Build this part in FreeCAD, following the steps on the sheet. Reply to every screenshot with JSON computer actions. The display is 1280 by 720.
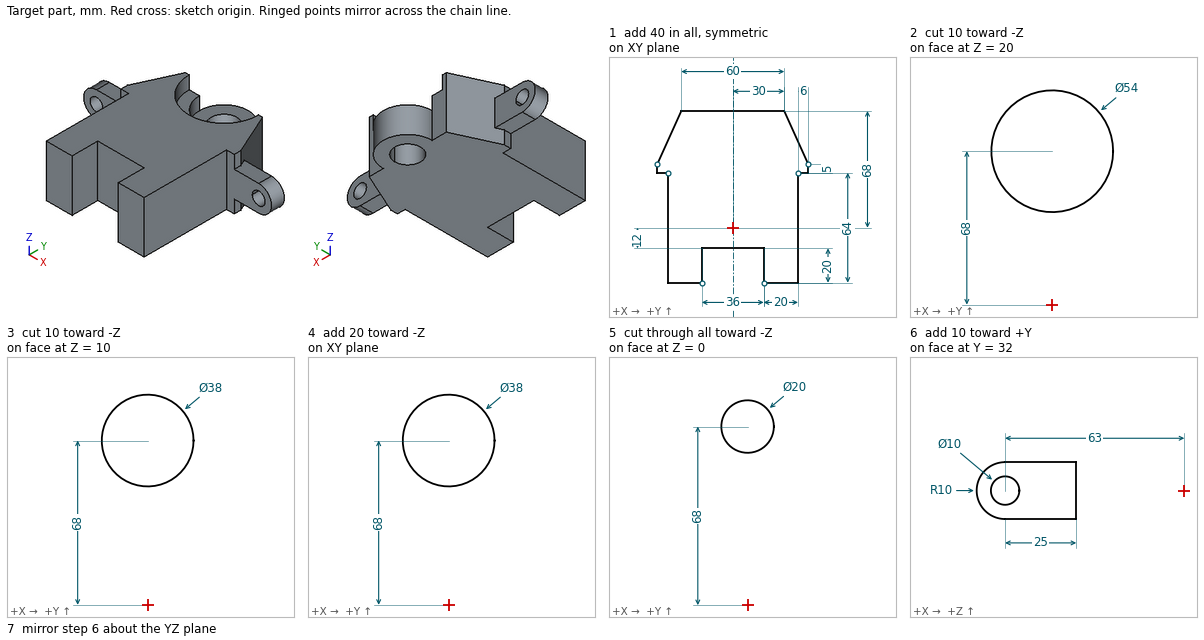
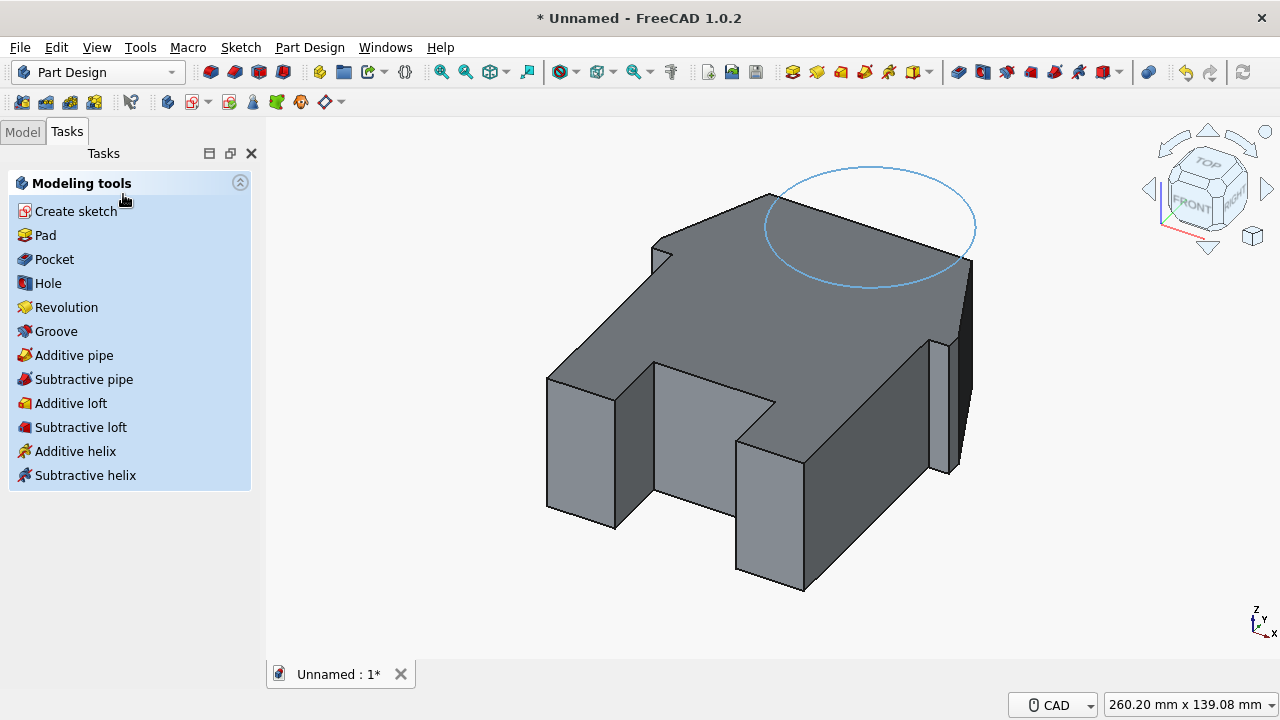
{"action": "left_click", "coordinate": [960, 72]}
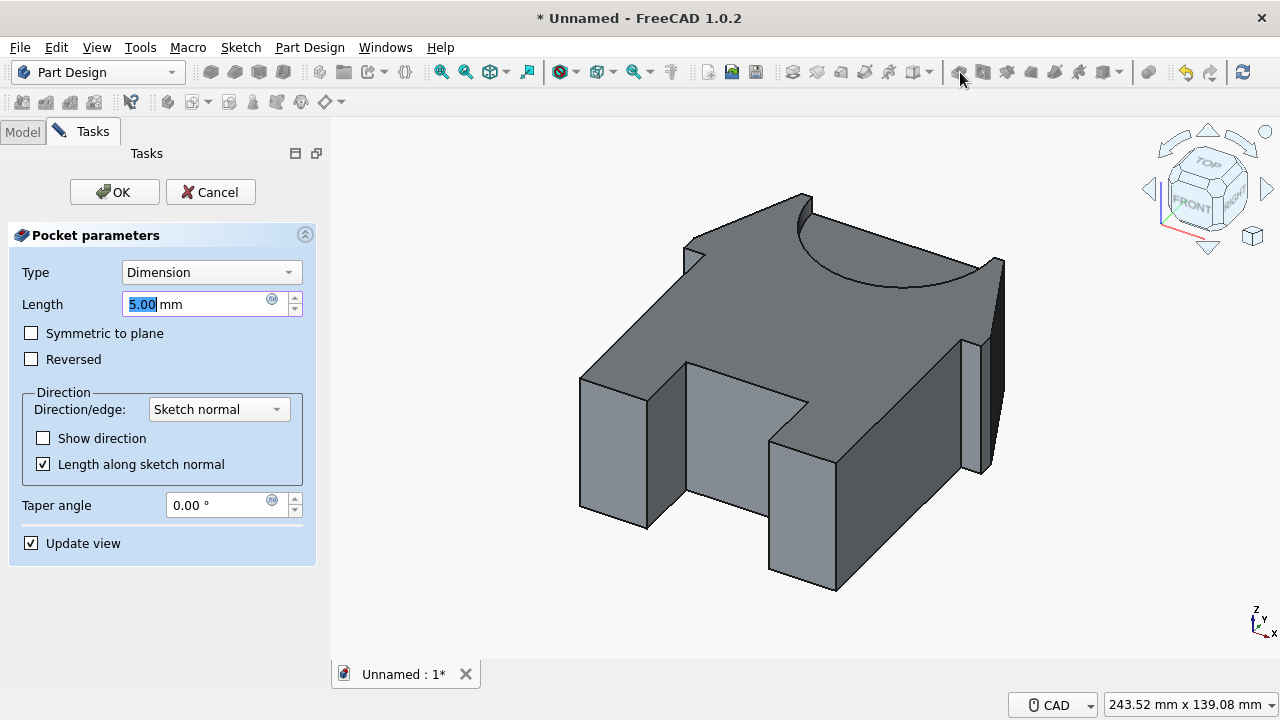
{"action": "type", "text": "10"}
{"action": "key", "text": "Tab"}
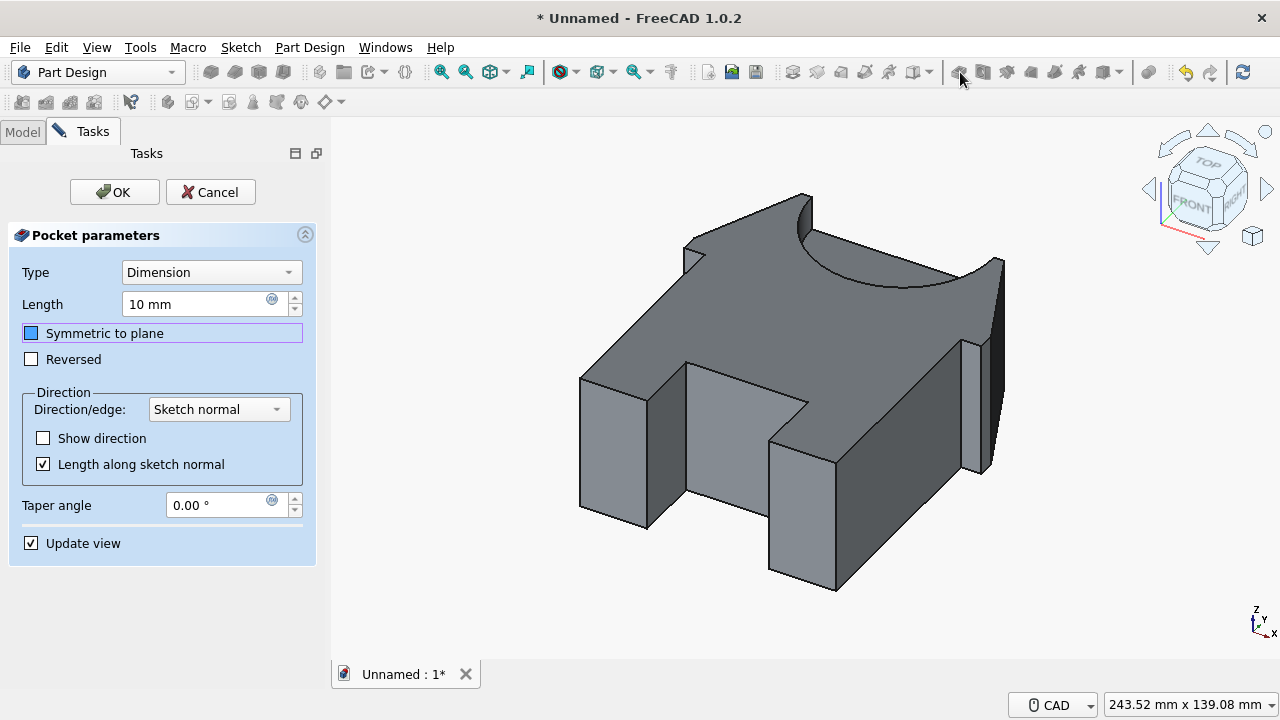
{"action": "left_click", "coordinate": [115, 192]}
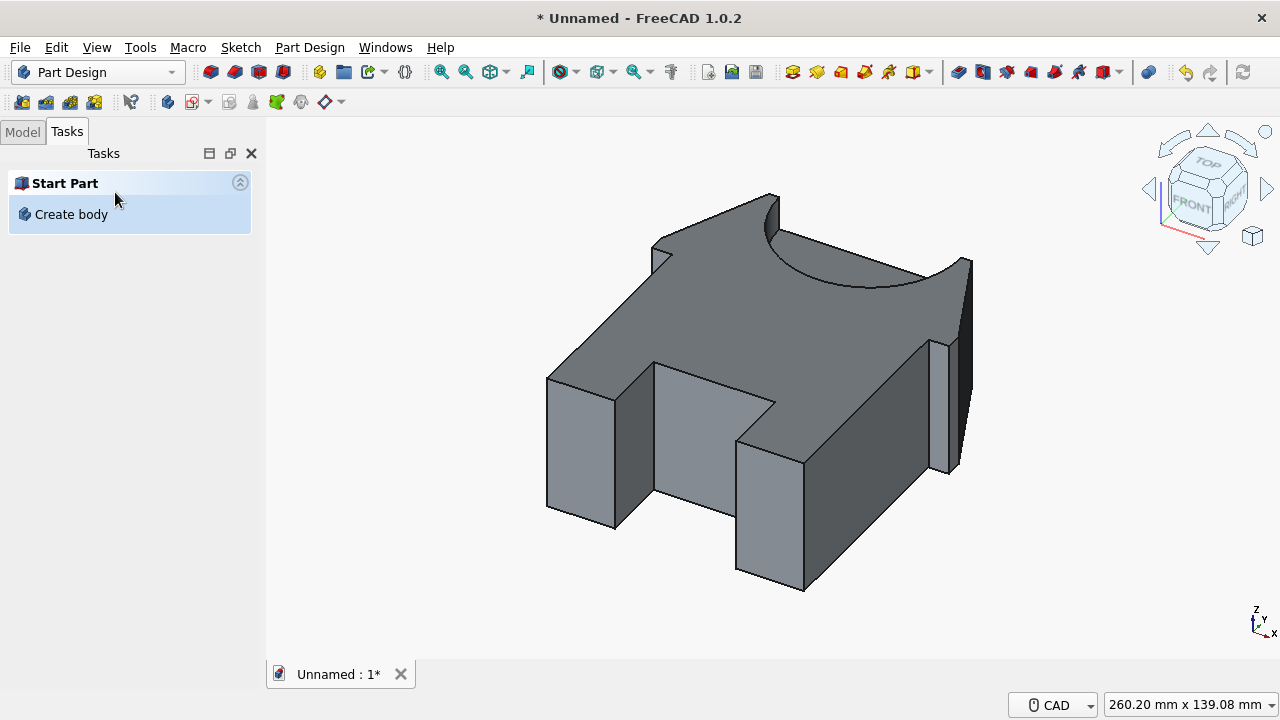
{"action": "left_click", "coordinate": [852, 277]}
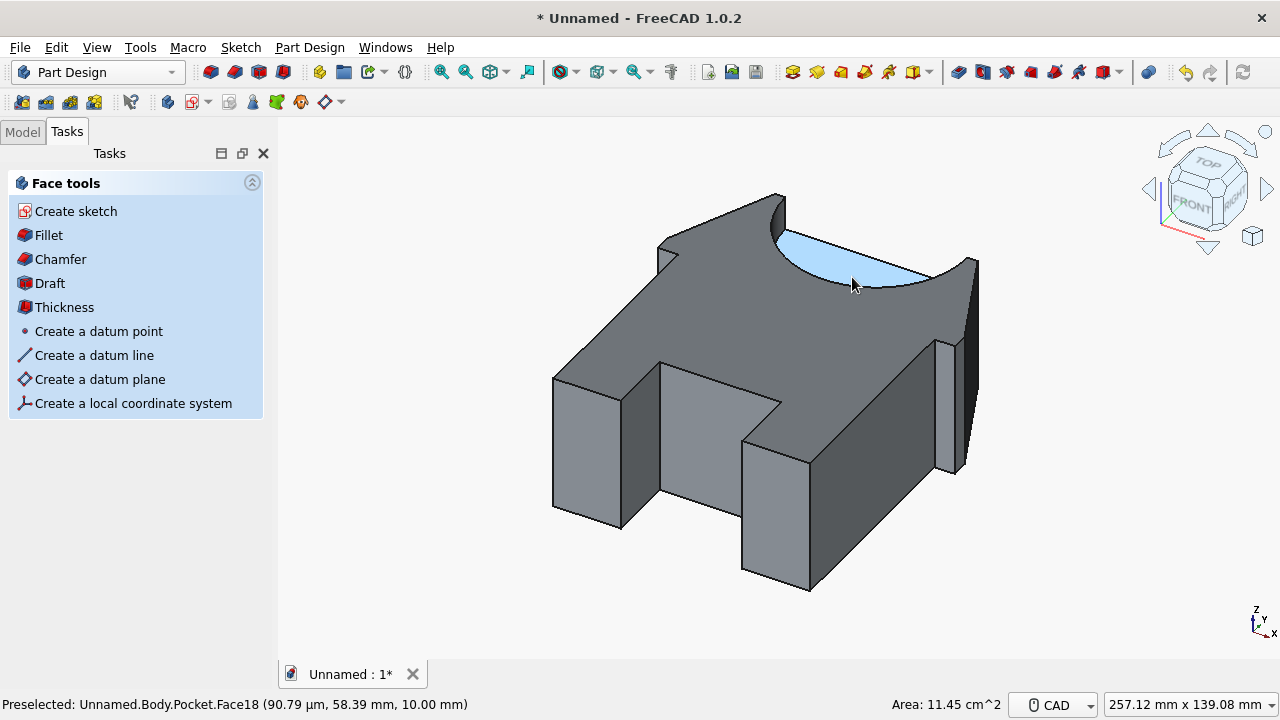
{"action": "left_click", "coordinate": [192, 102]}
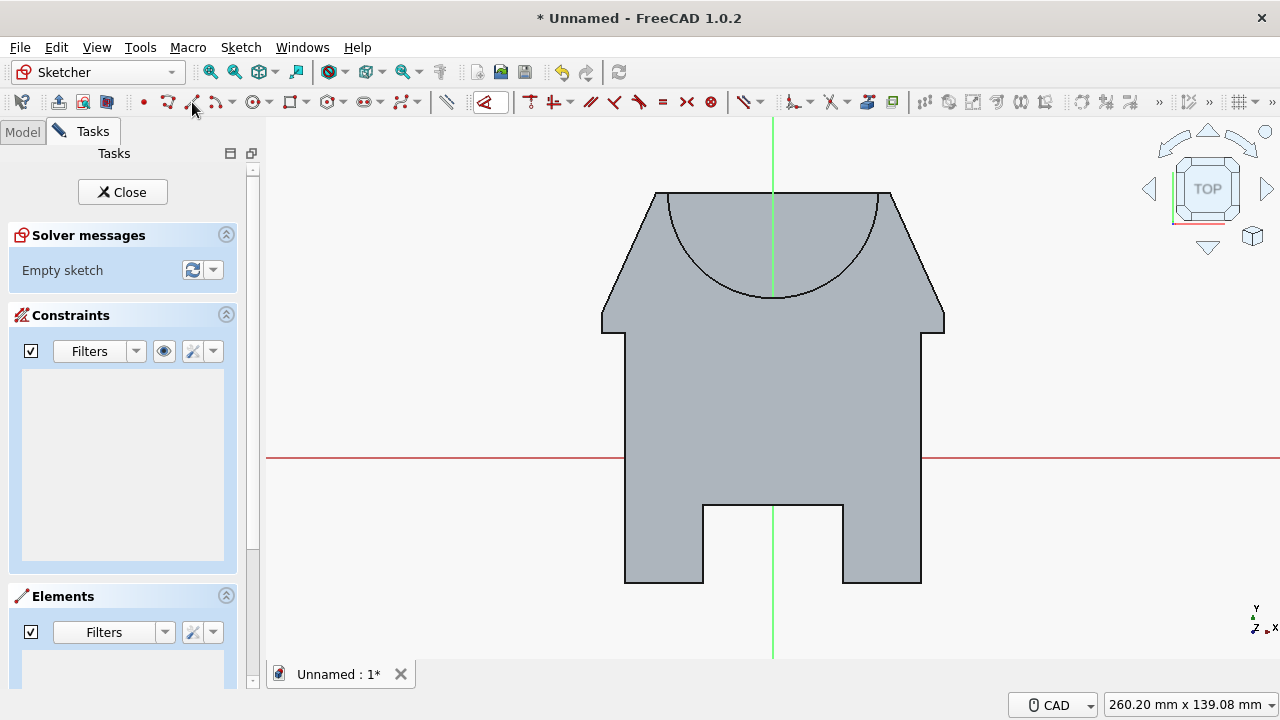
{"action": "left_click", "coordinate": [108, 102]}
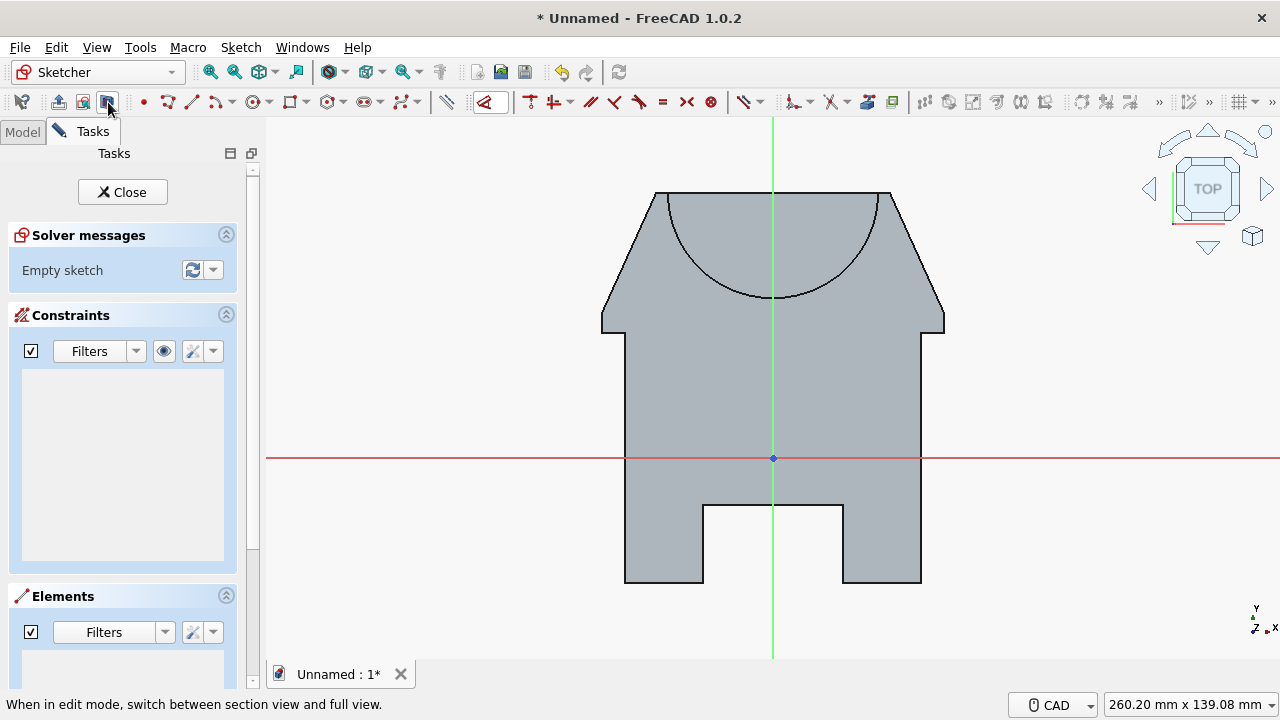
{"action": "scroll", "coordinate": [395, 631], "scroll_direction": "down", "scroll_amount": 1}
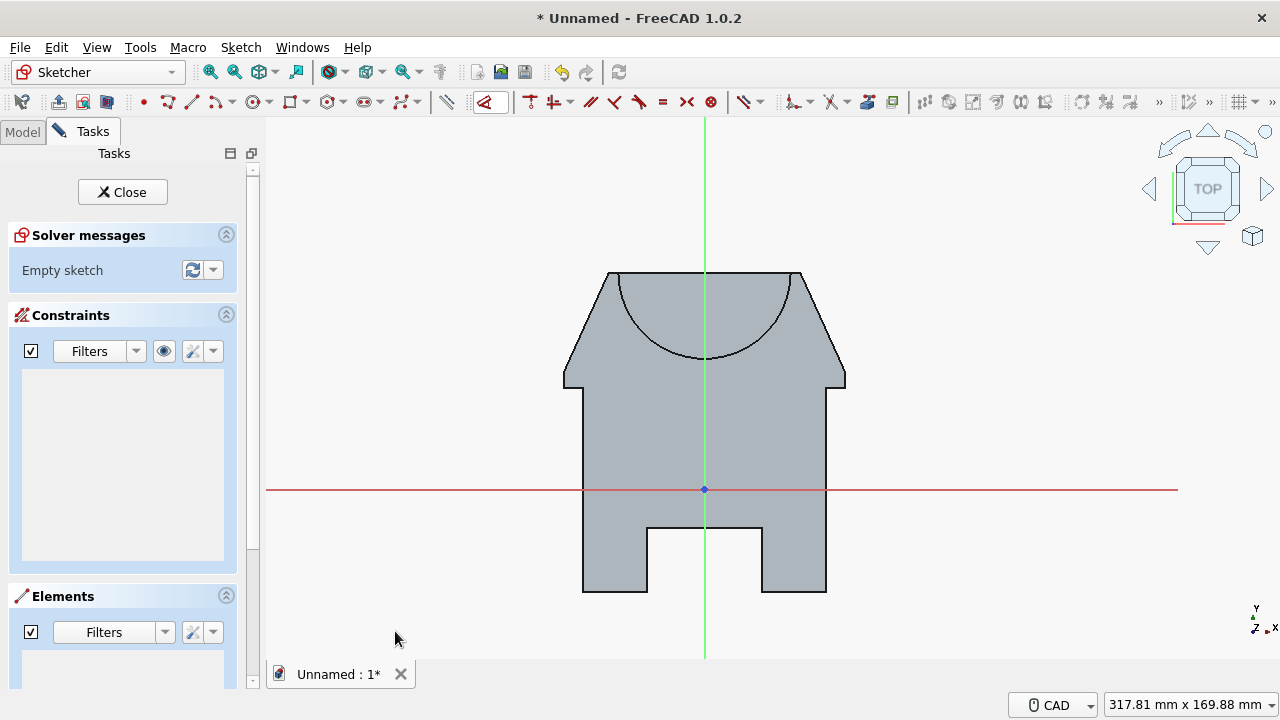
{"action": "left_click", "coordinate": [254, 102]}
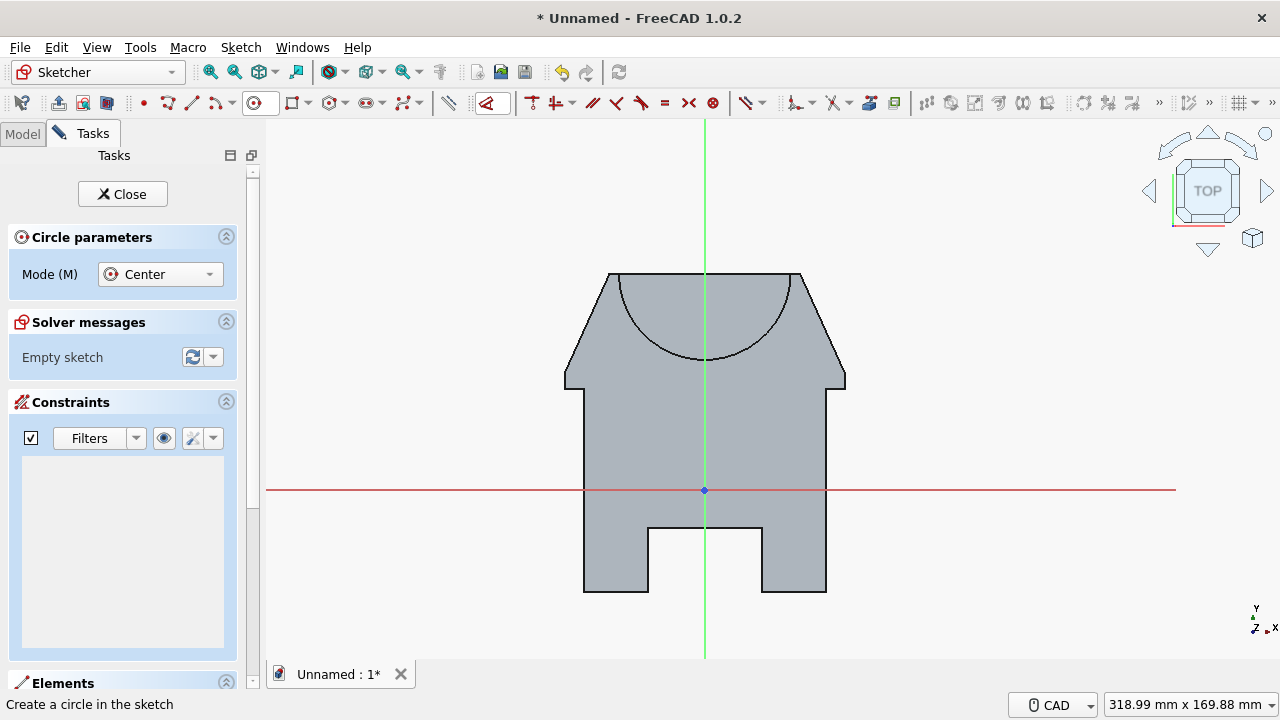
{"action": "left_click", "coordinate": [705, 274]}
{"action": "left_click", "coordinate": [747, 231]}
{"action": "key", "text": "Escape"}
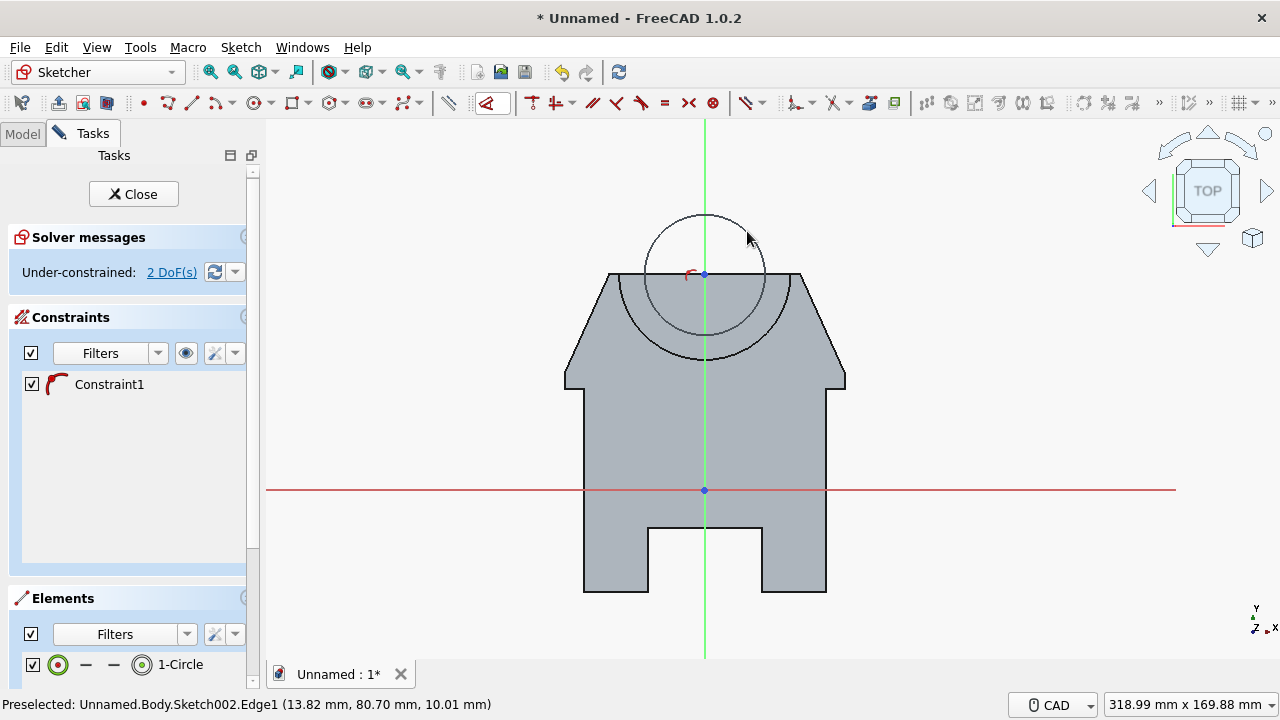
{"action": "left_click", "coordinate": [747, 232]}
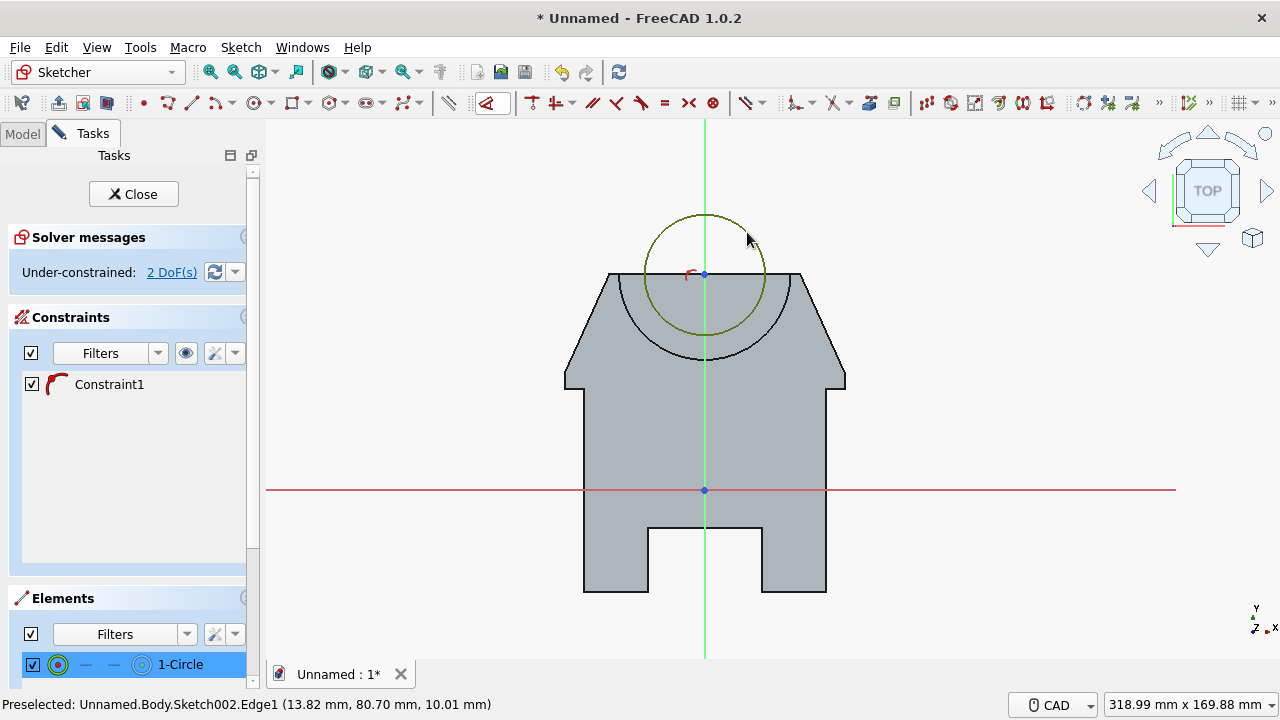
{"action": "left_click", "coordinate": [504, 104]}